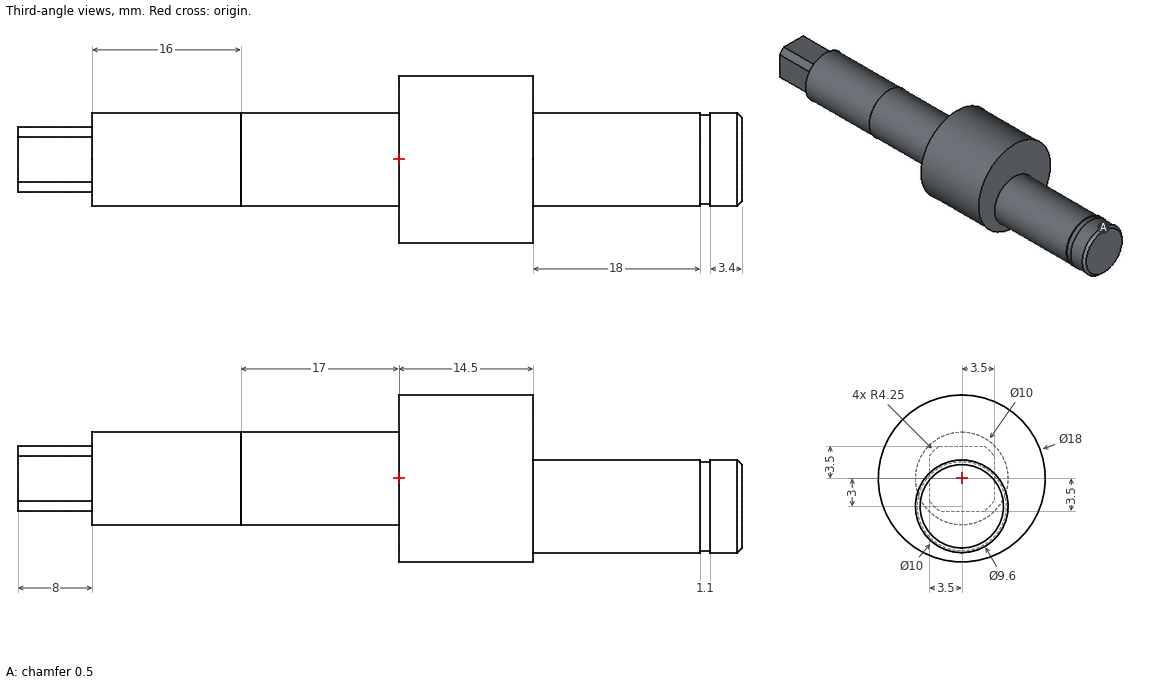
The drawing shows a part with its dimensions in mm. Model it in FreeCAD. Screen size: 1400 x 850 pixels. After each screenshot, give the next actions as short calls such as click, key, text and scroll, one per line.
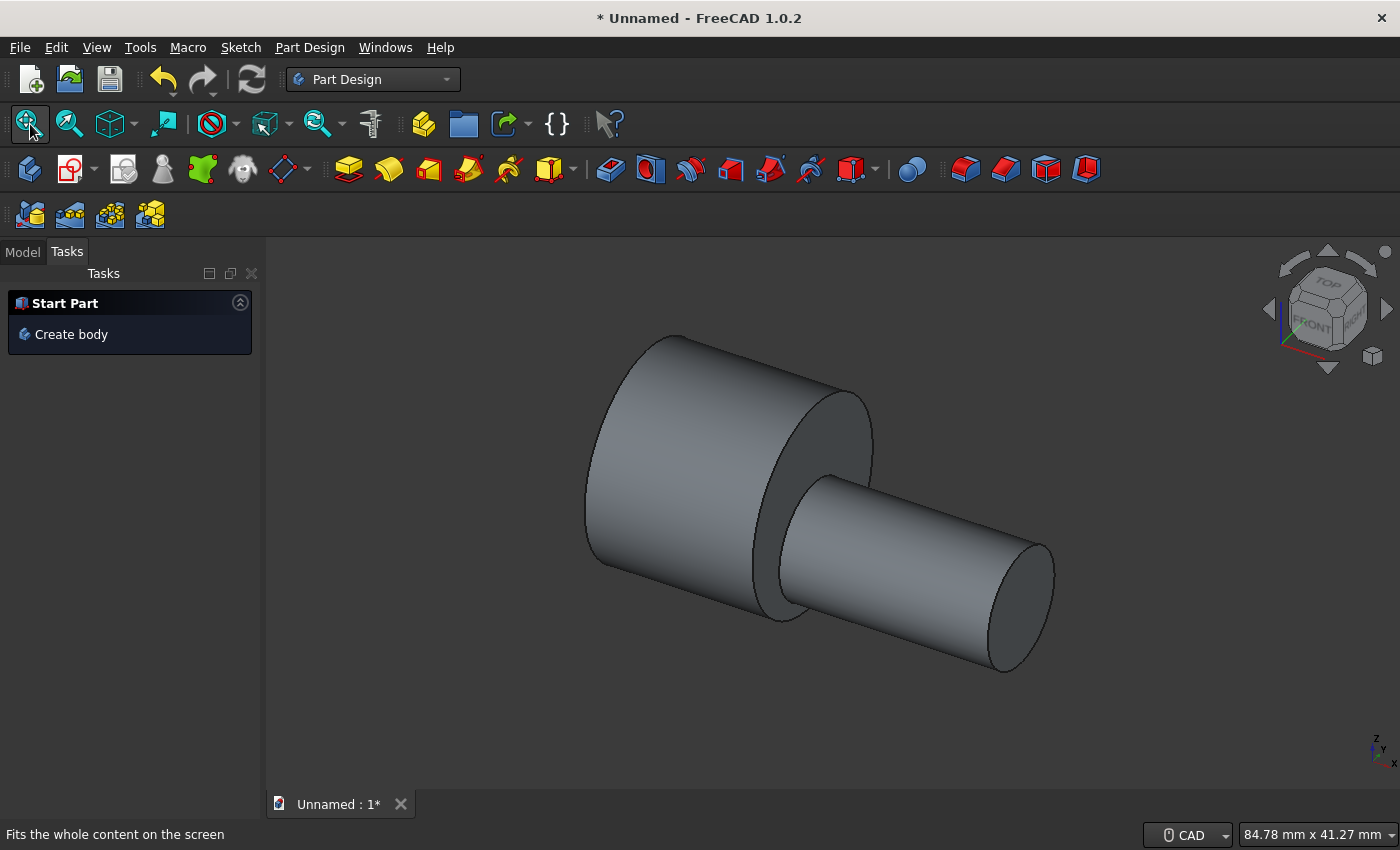
click(1021, 607)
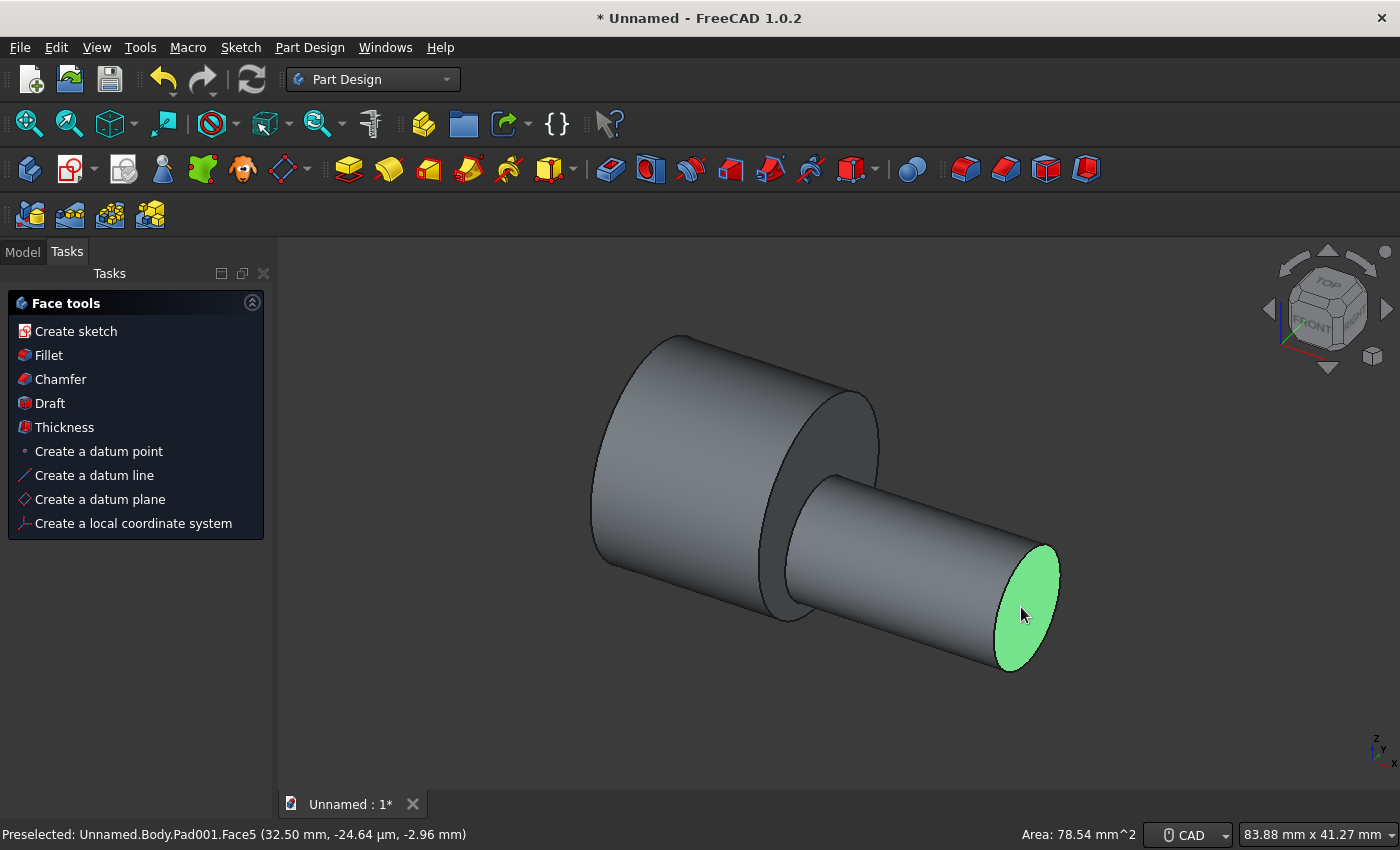
click(70, 170)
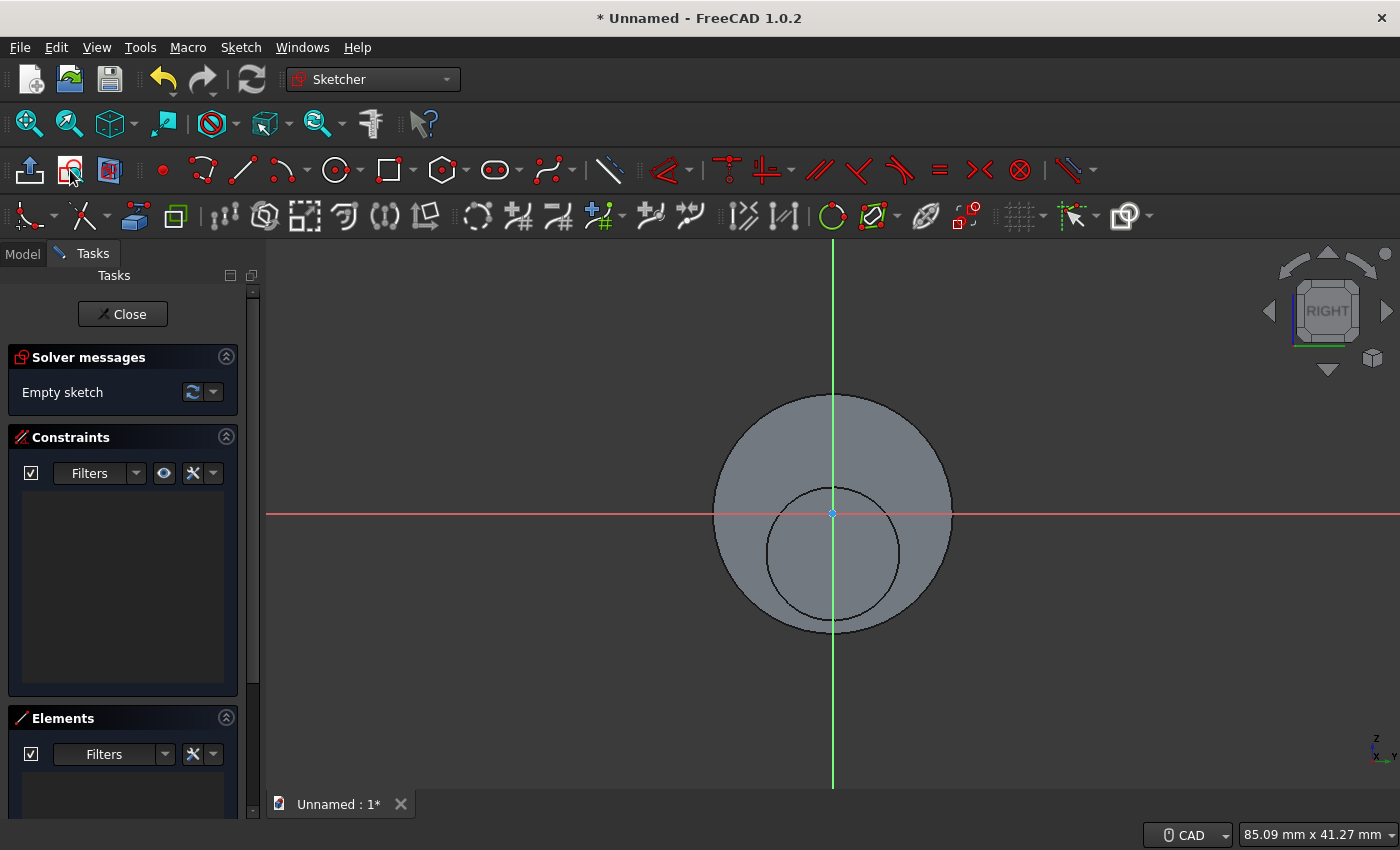
scroll(873, 577, up, 5)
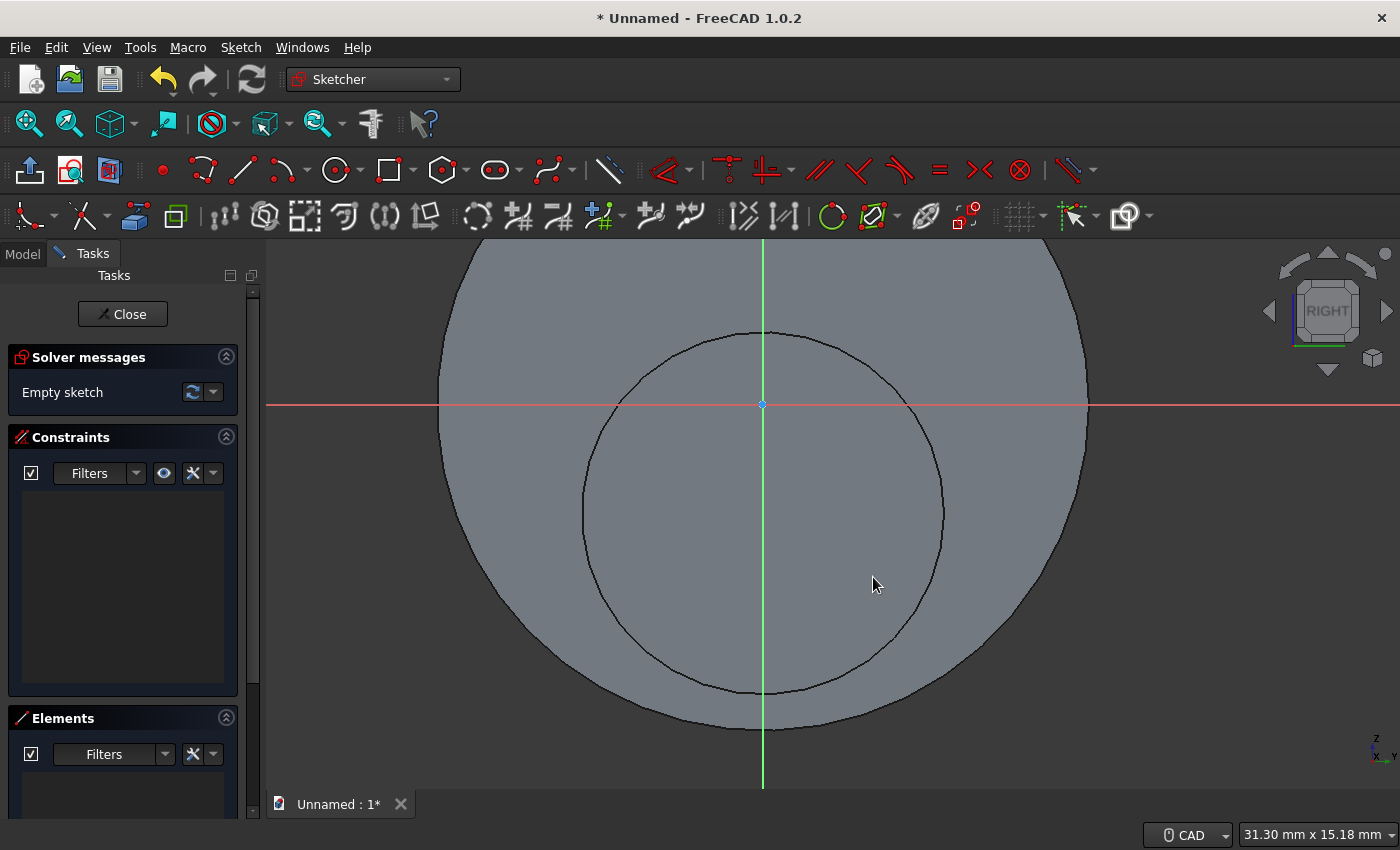
click(336, 170)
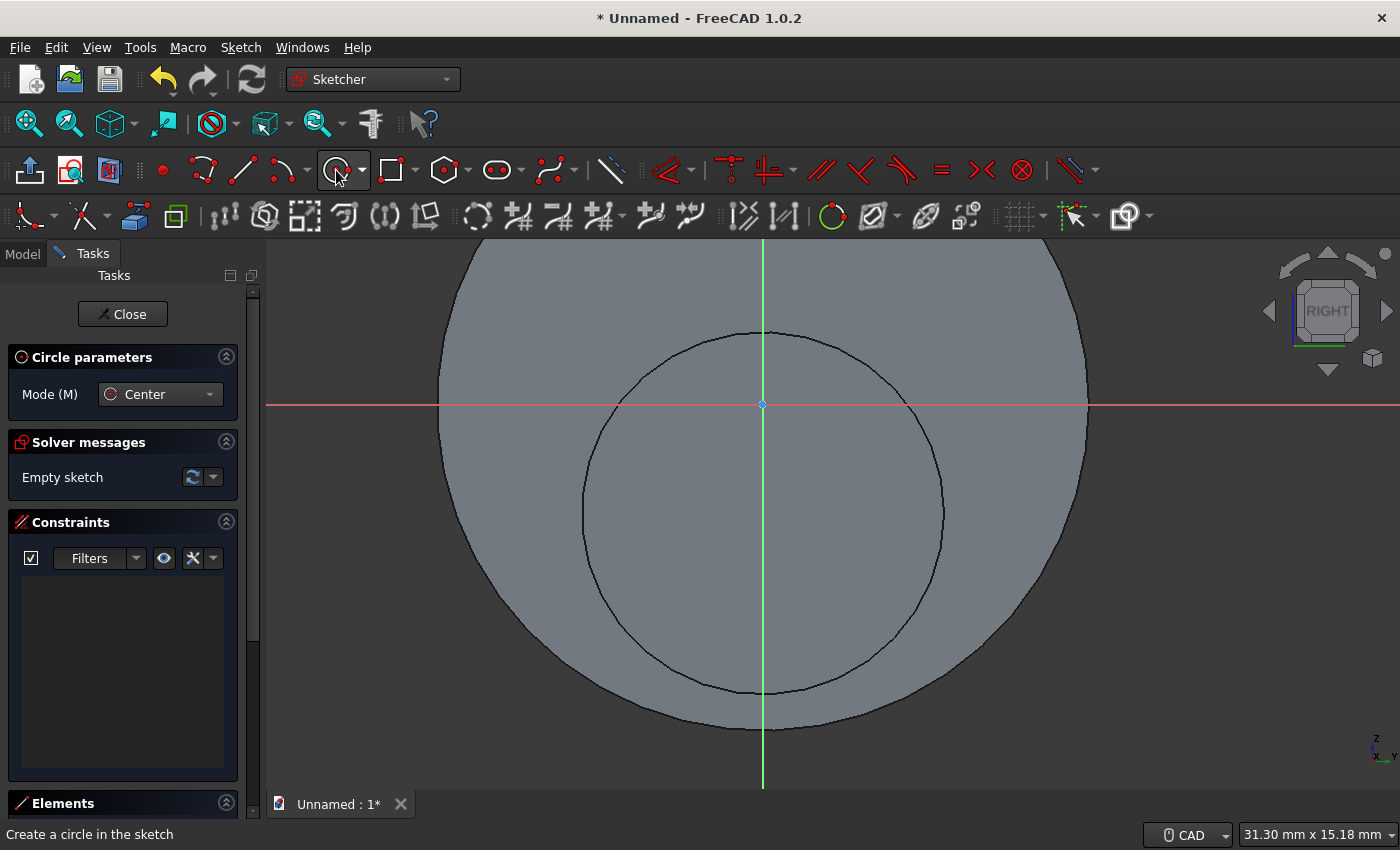
click(763, 513)
move(886, 390)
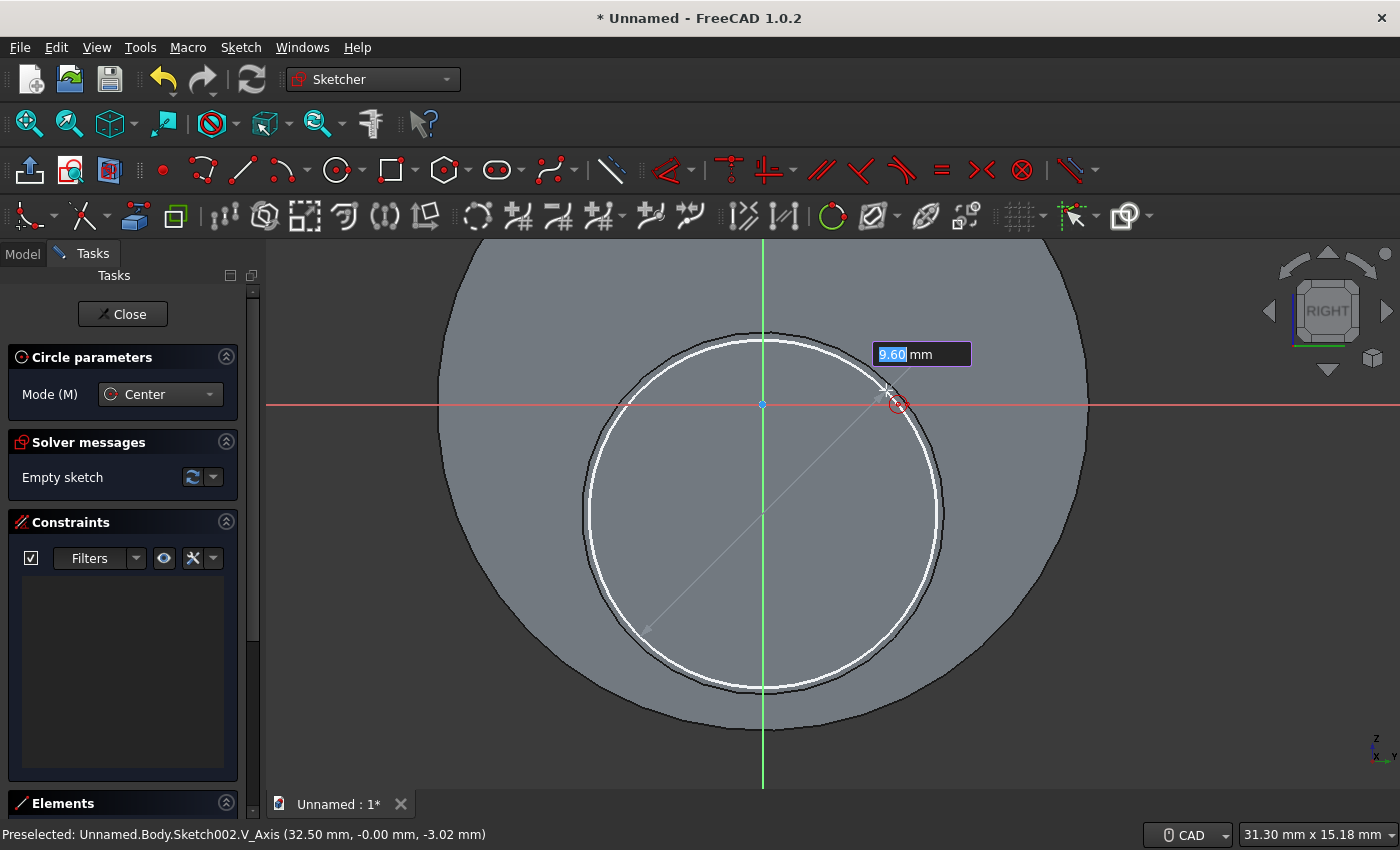
text(9.6)
key(Return)
key(Escape)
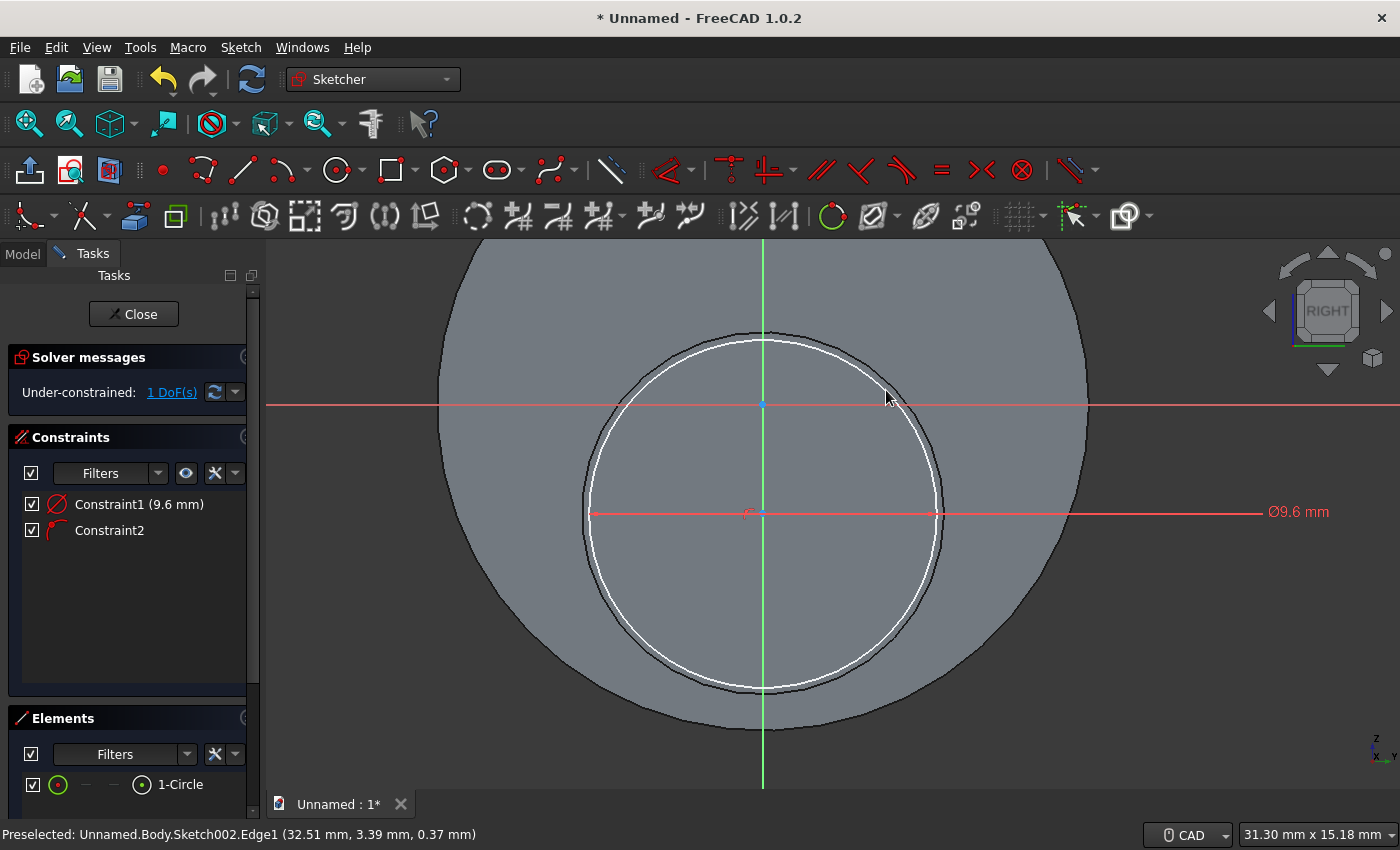
click(666, 170)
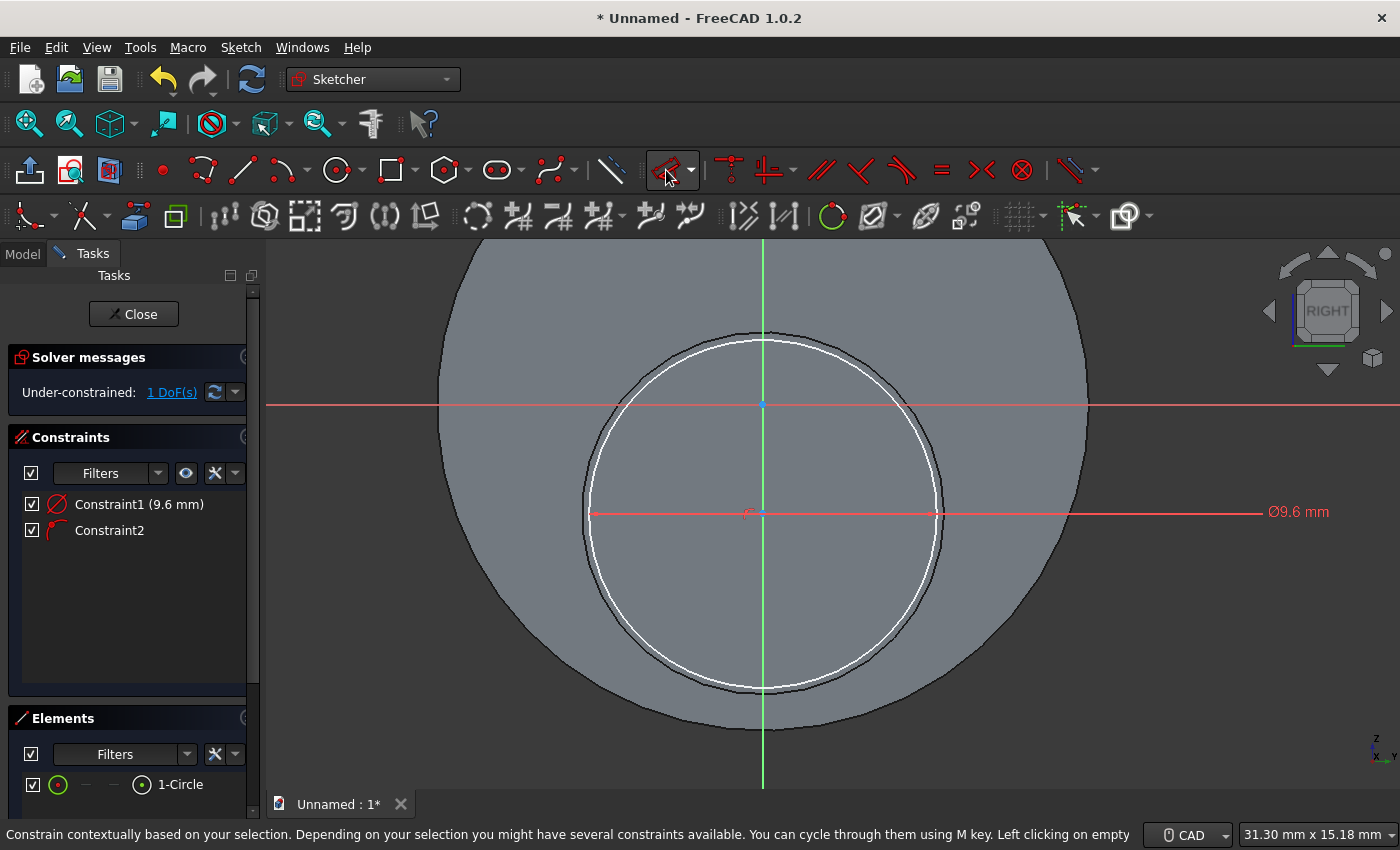
click(763, 514)
click(797, 459)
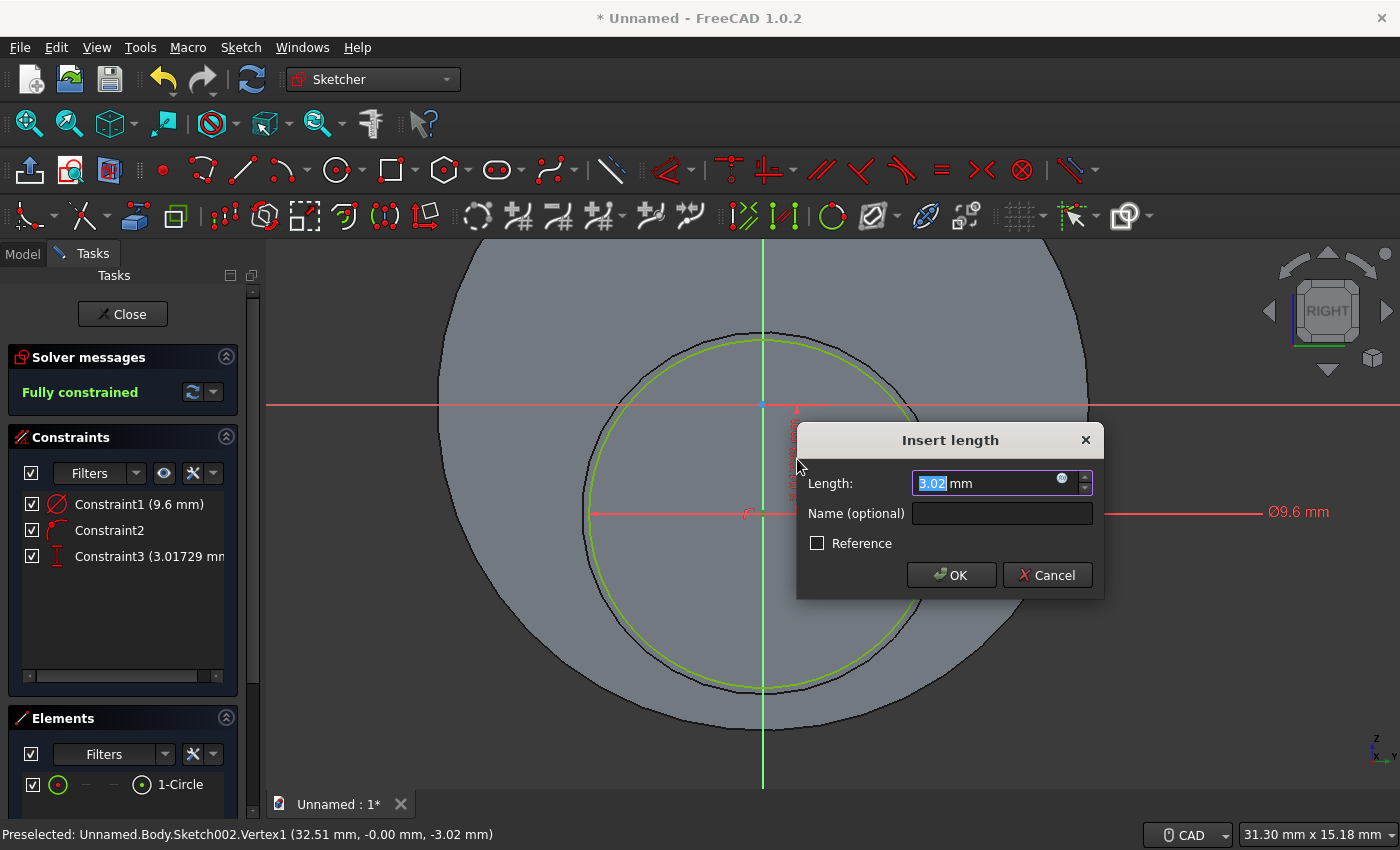
text(3)
key(Return)
key(Escape)